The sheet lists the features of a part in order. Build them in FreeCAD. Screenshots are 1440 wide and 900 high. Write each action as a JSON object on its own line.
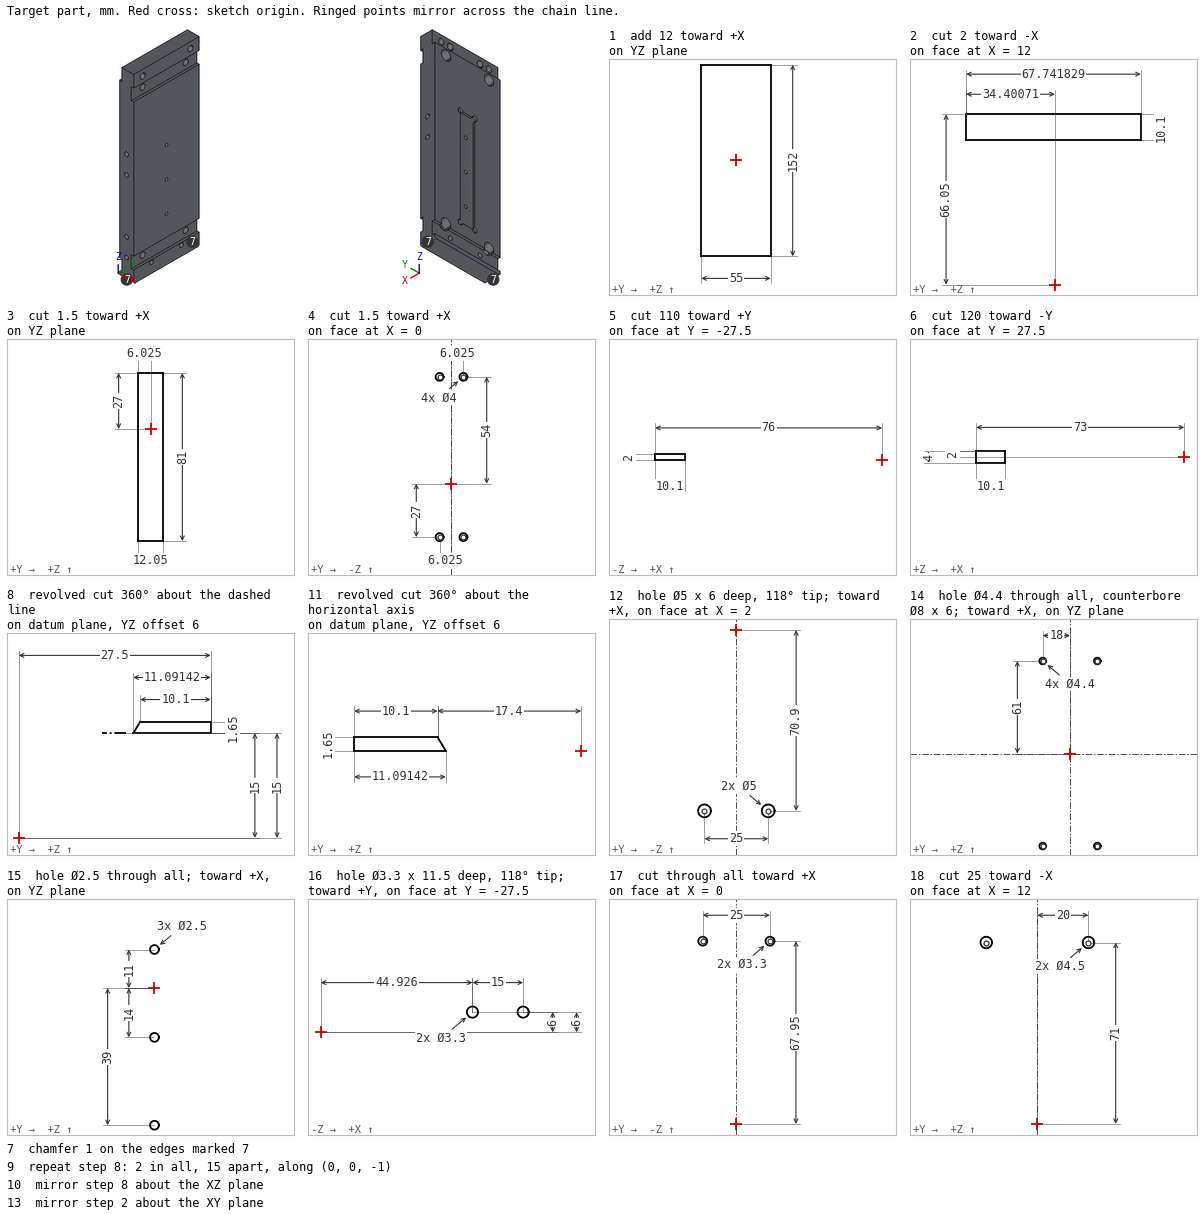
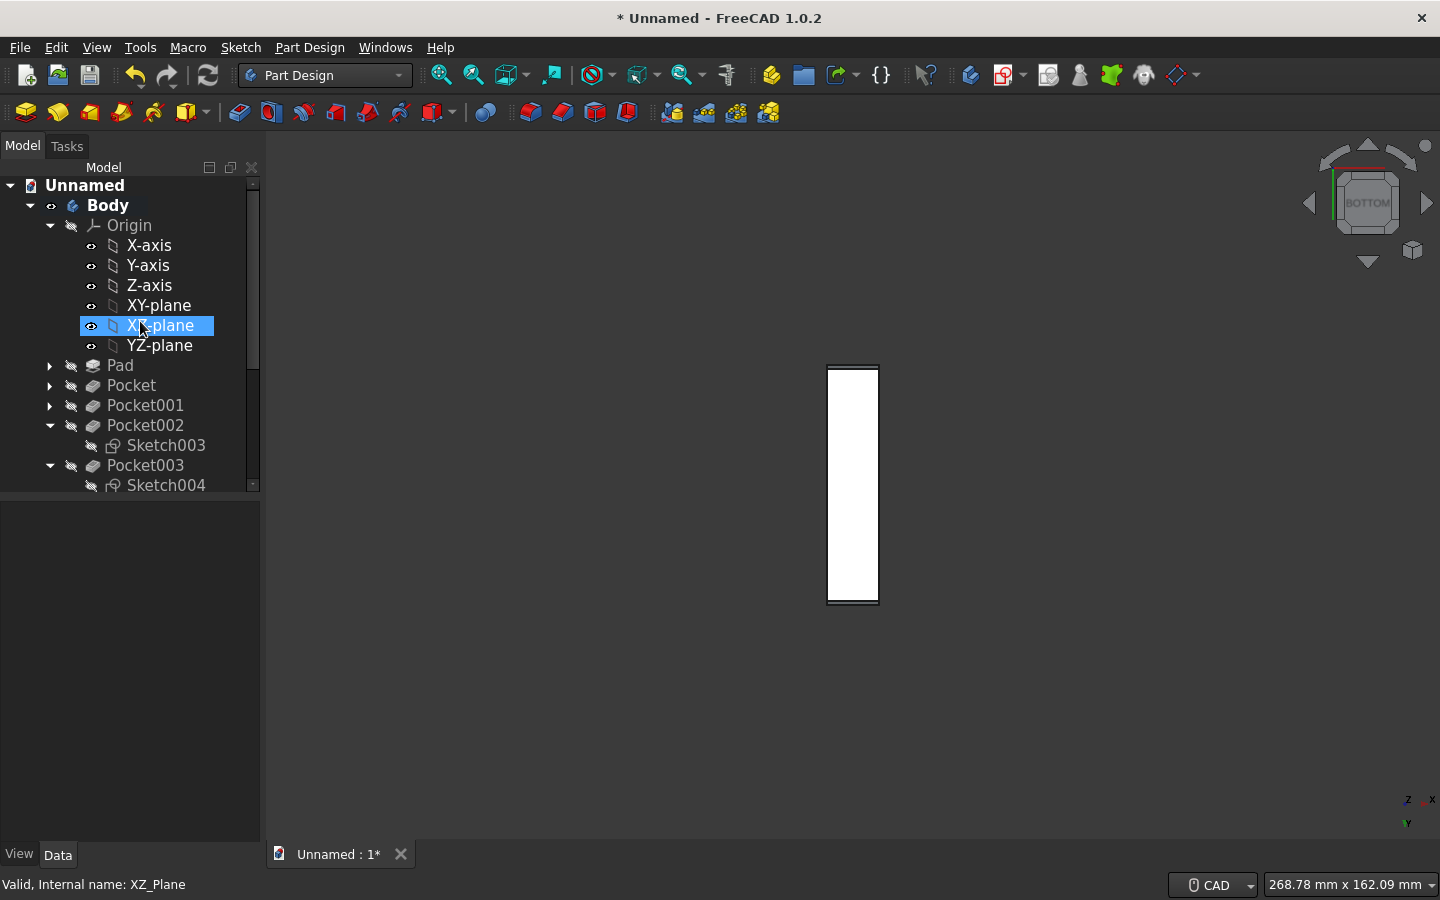
{"action": "left_click", "coordinate": [136, 346]}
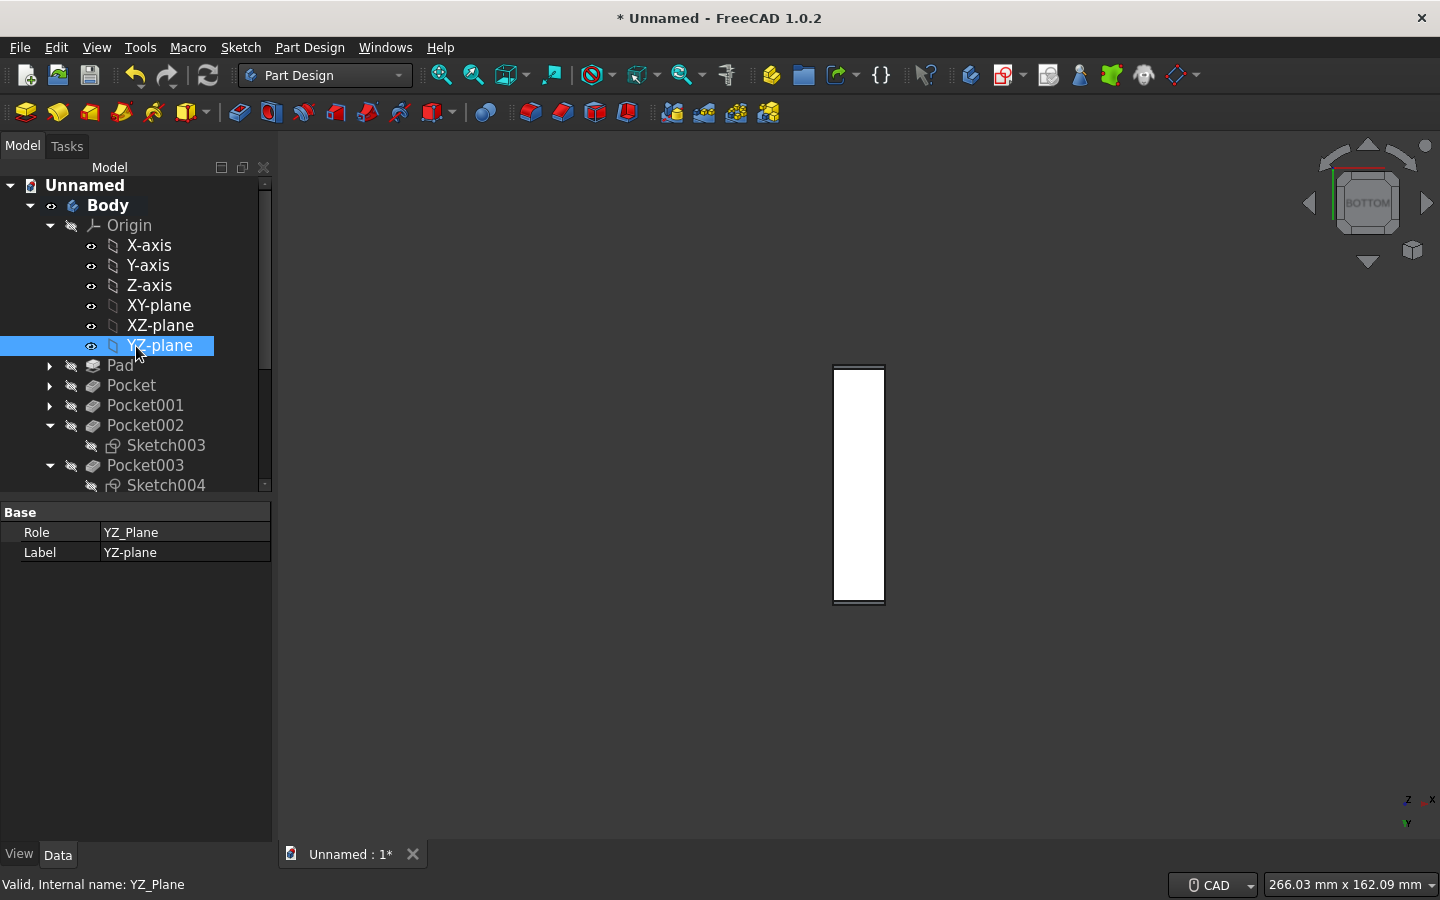
{"action": "left_click", "coordinate": [1176, 76]}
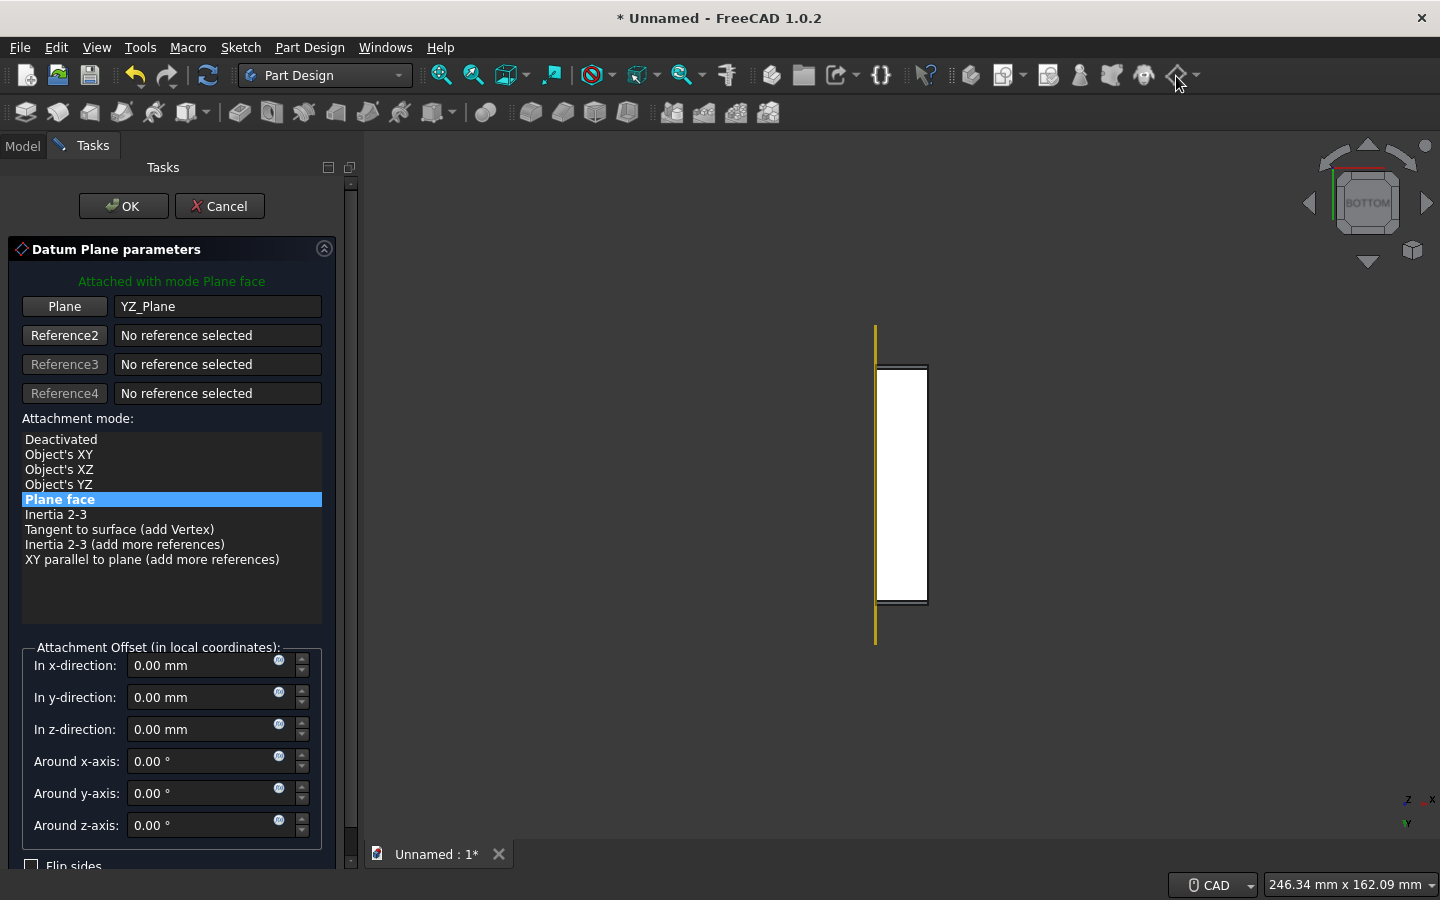
{"action": "triple_click", "coordinate": [210, 729]}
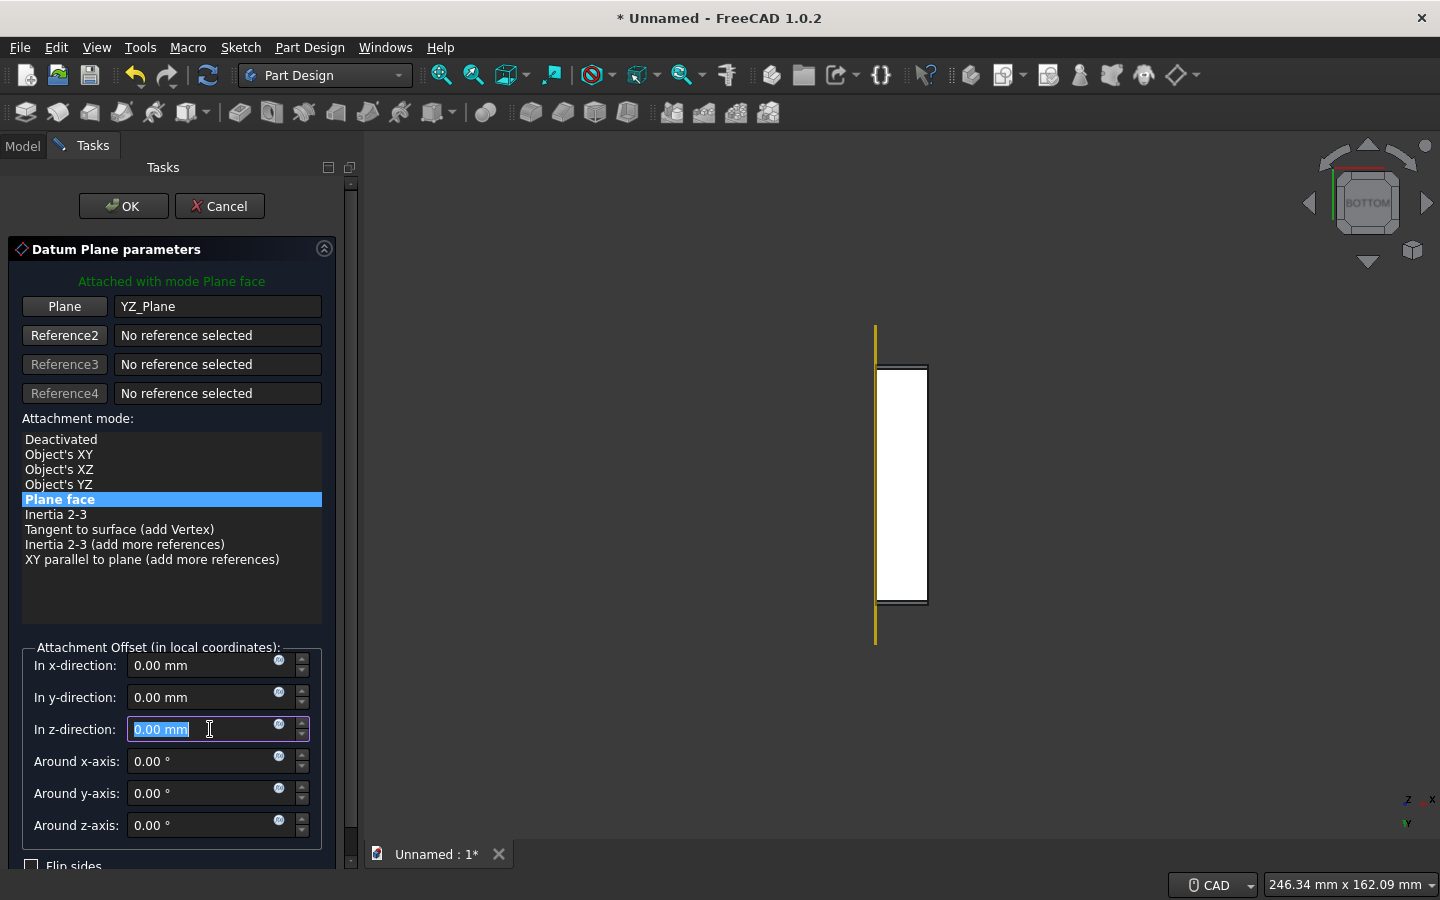
{"action": "type", "text": "6"}
{"action": "key", "text": "Tab"}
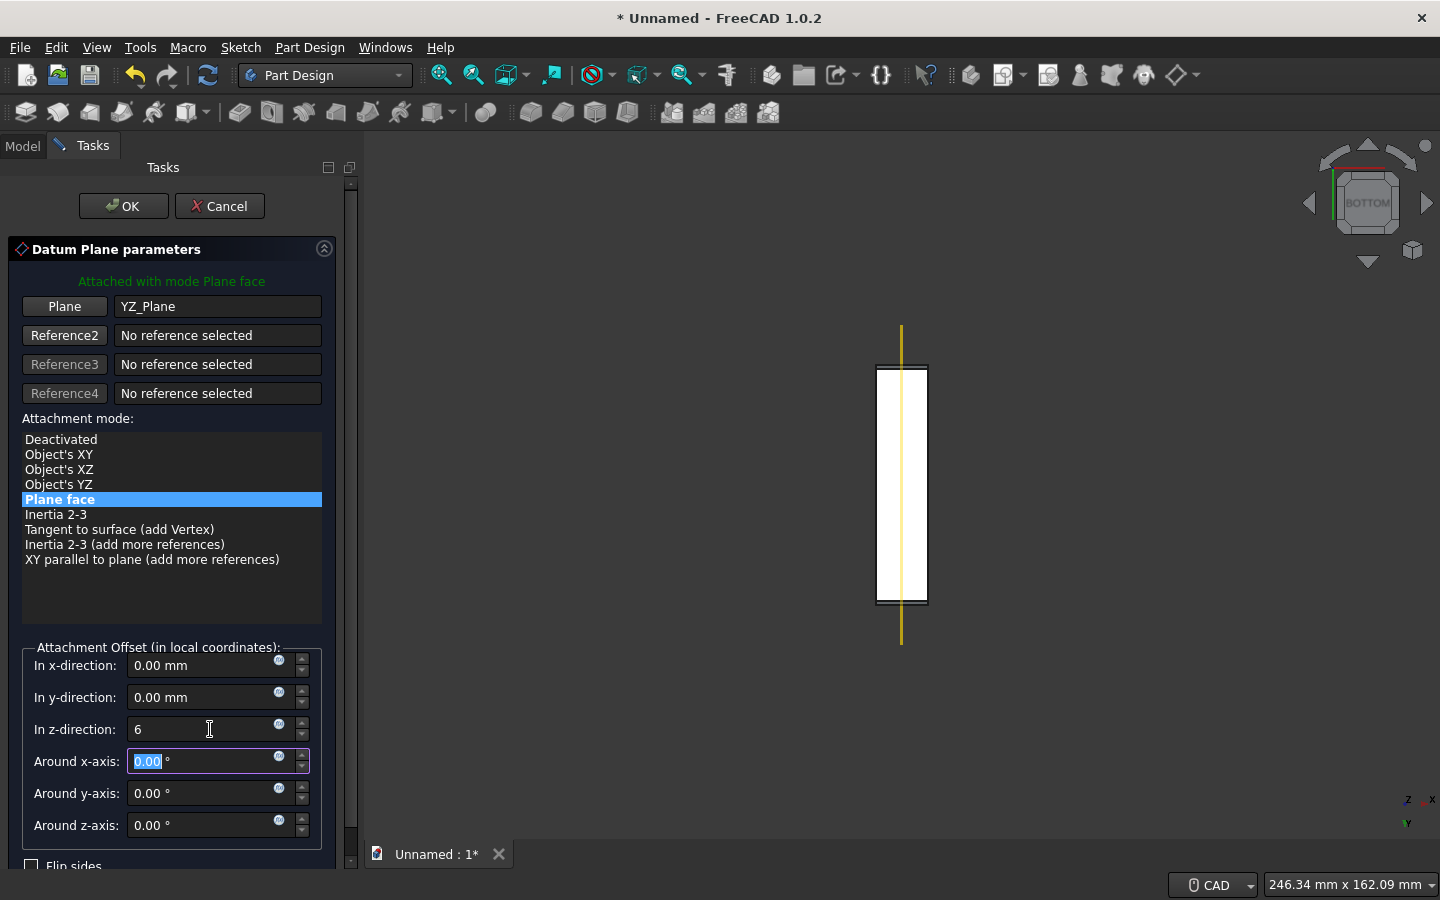
{"action": "left_click", "coordinate": [124, 206]}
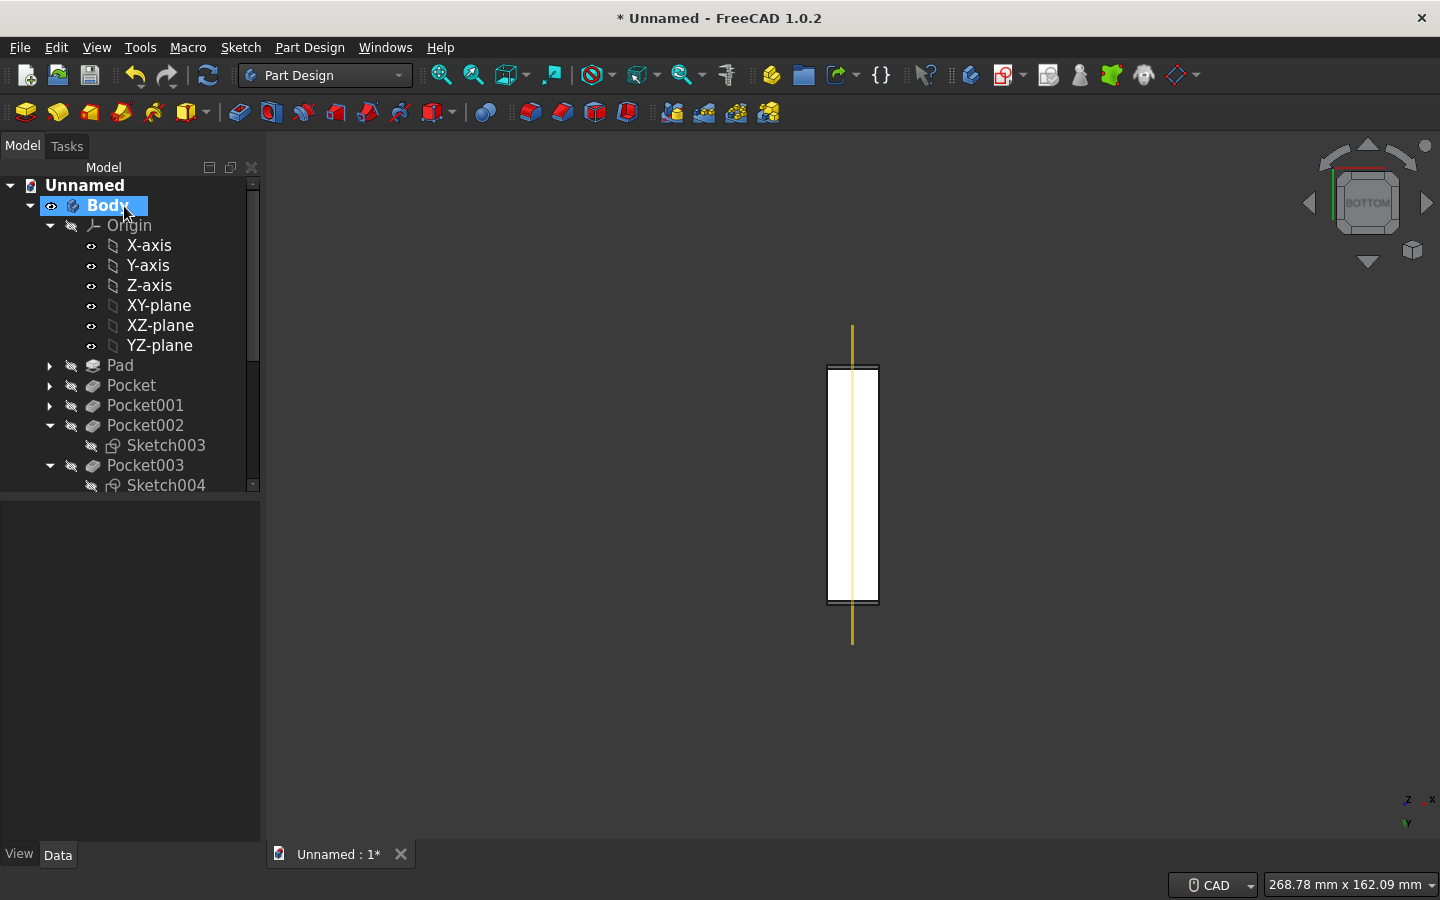
{"action": "scroll", "coordinate": [100, 341], "scroll_direction": "down", "scroll_amount": 3}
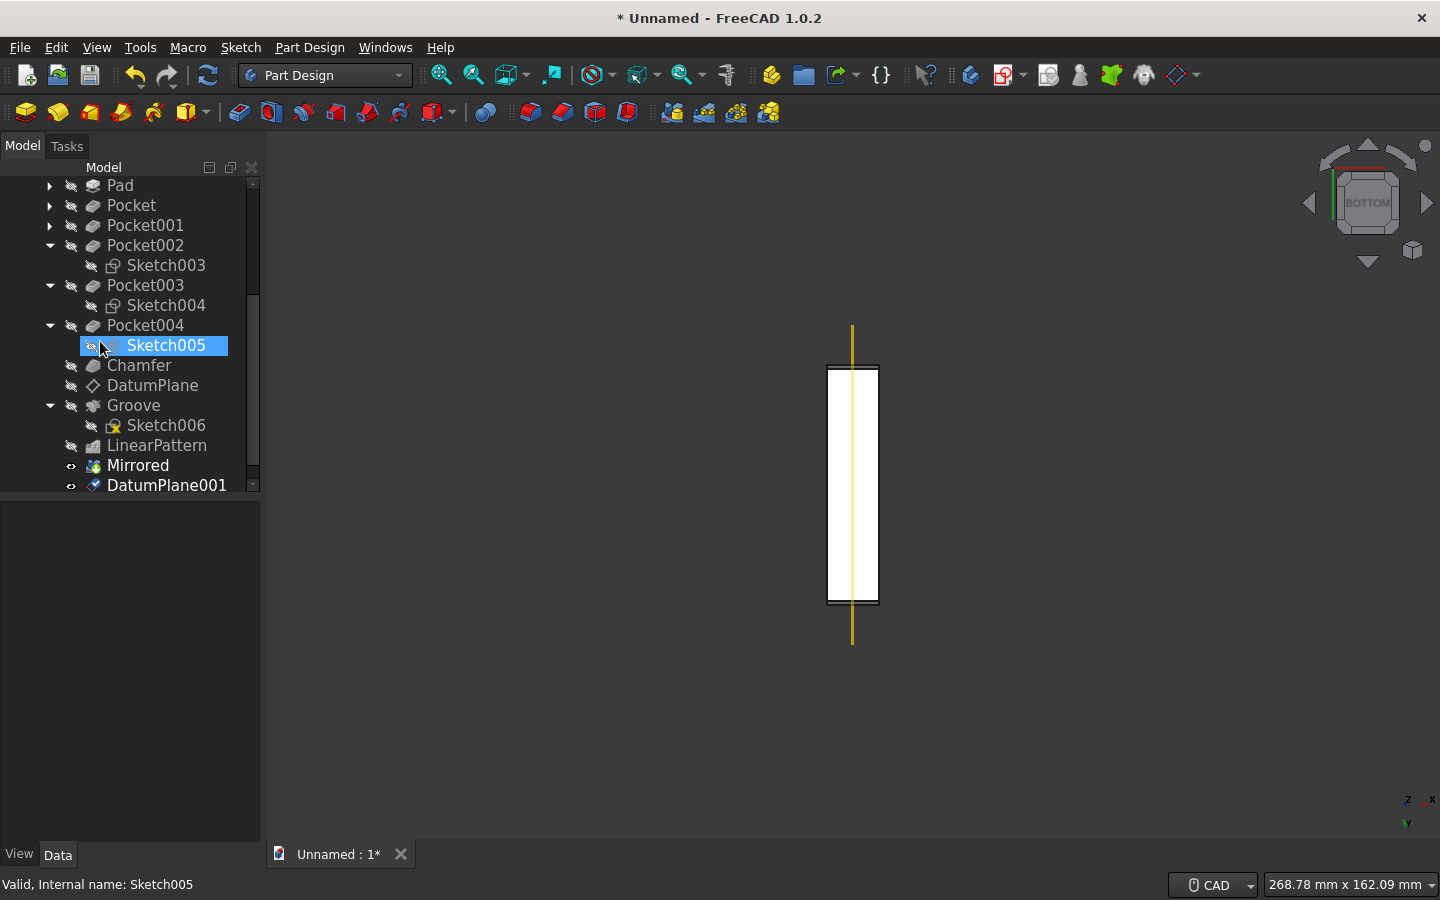
{"action": "left_click", "coordinate": [116, 486]}